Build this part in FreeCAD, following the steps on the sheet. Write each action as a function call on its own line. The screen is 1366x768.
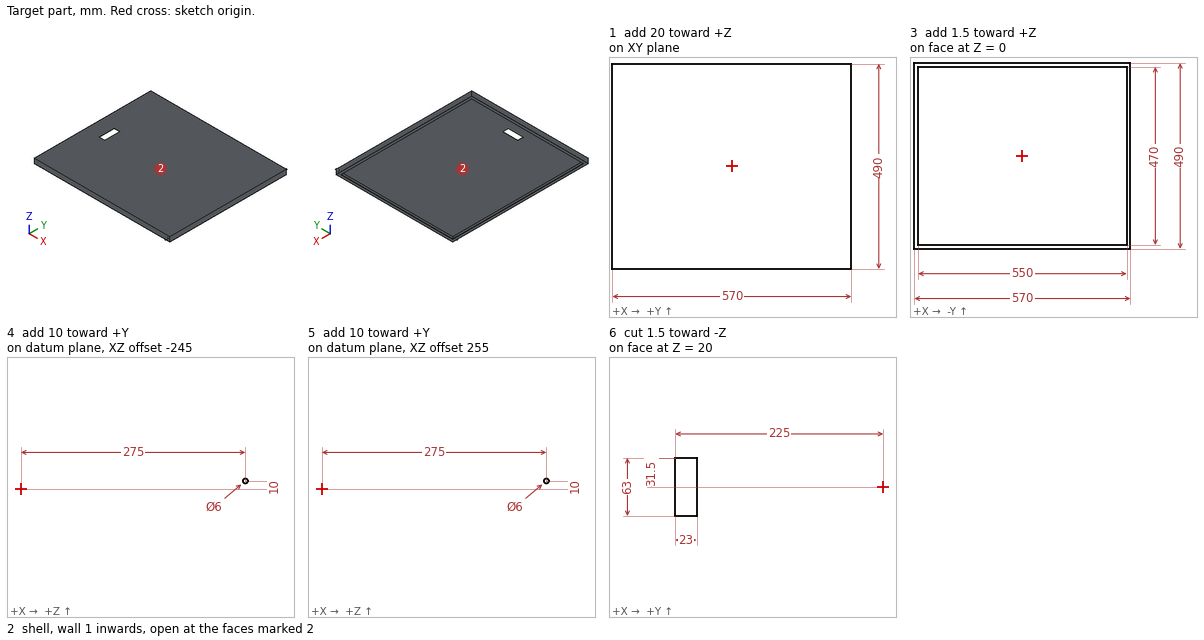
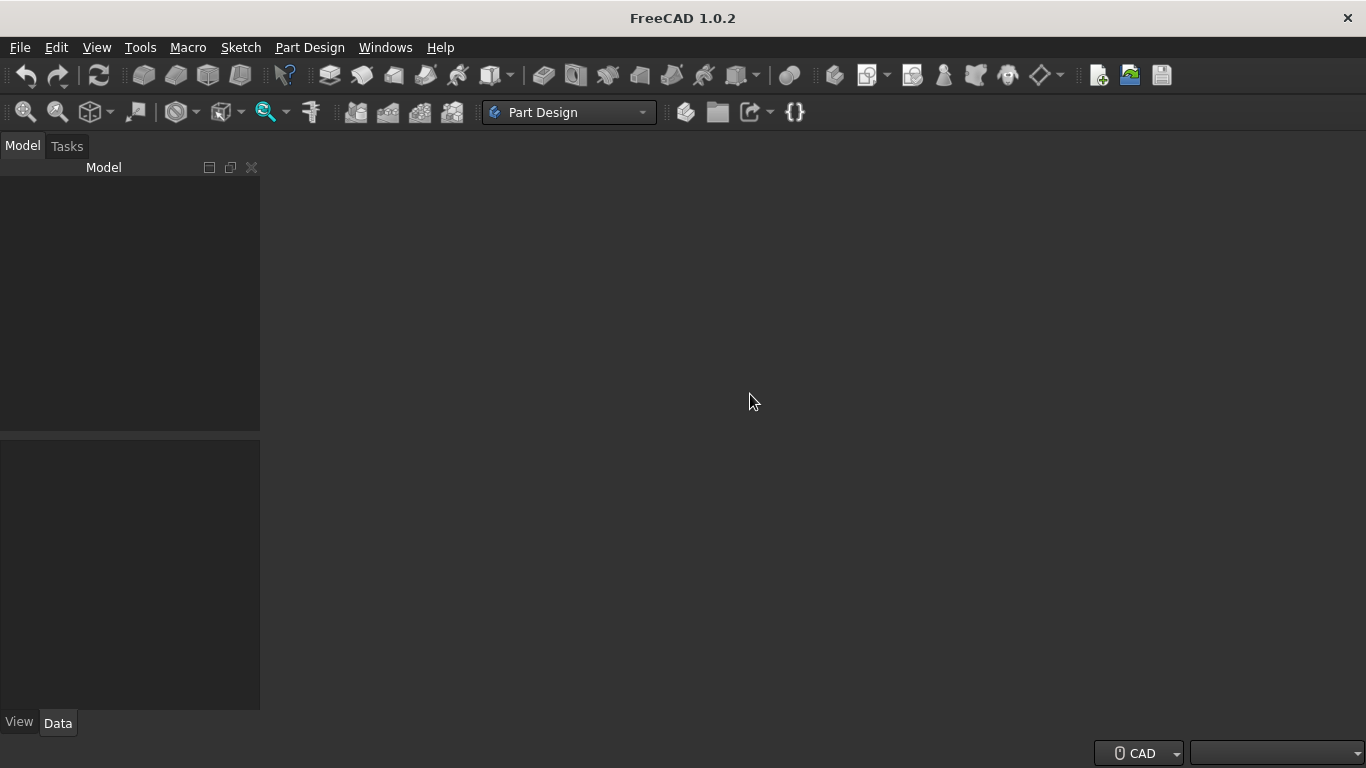
click(1098, 76)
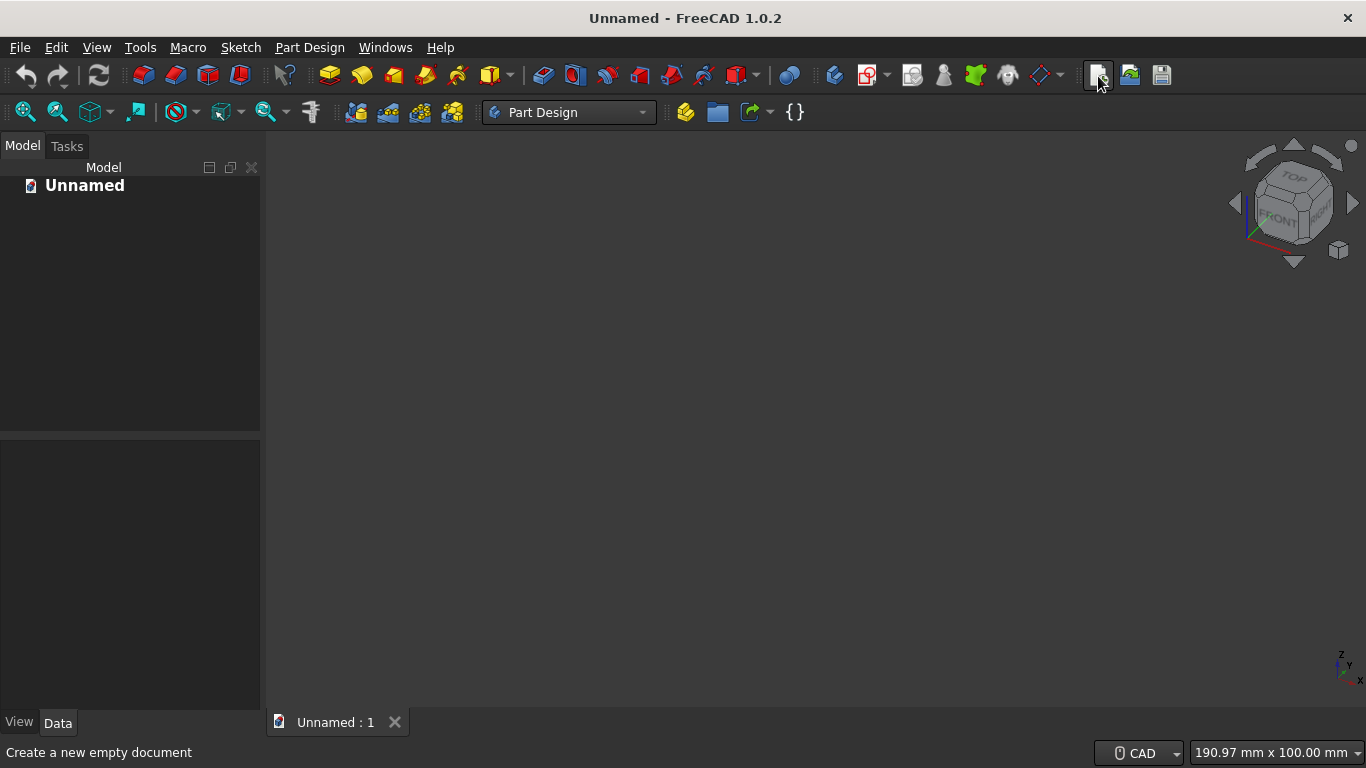
click(868, 76)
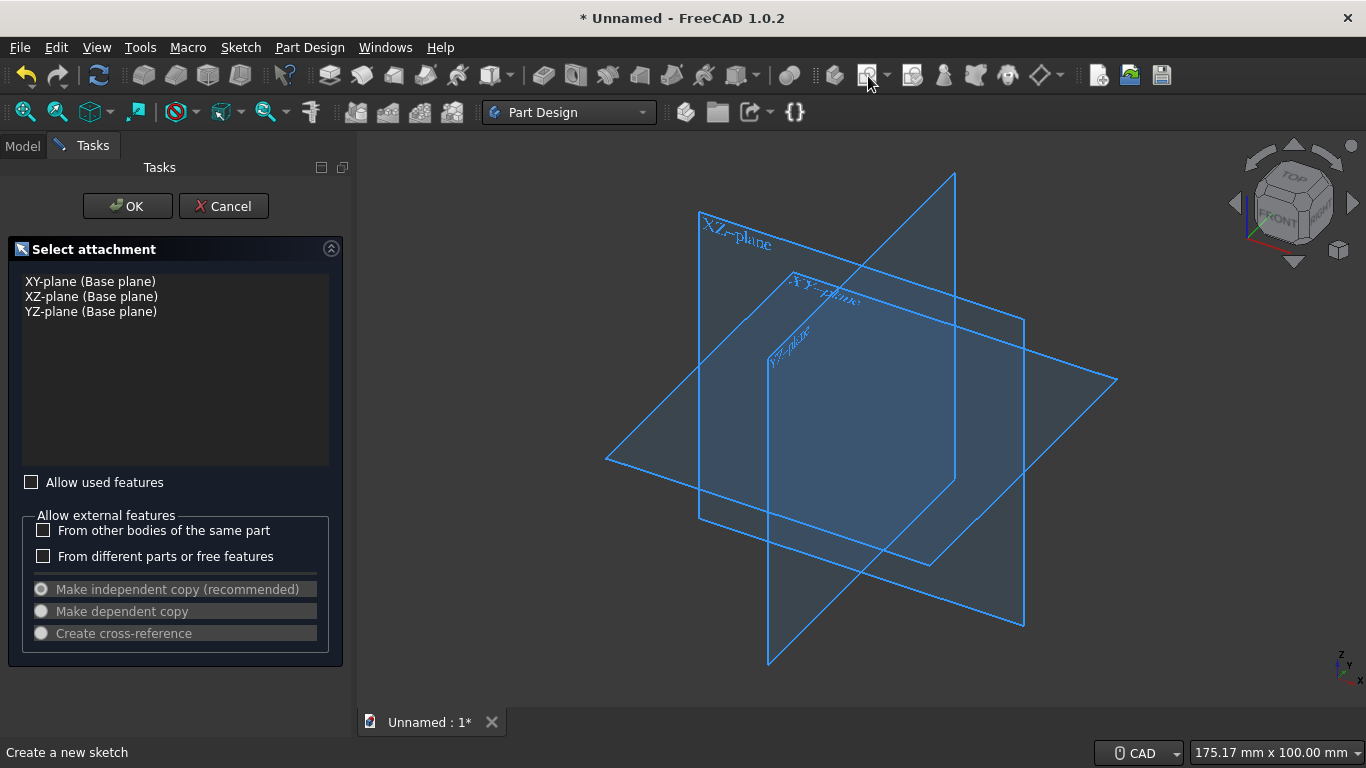
click(82, 282)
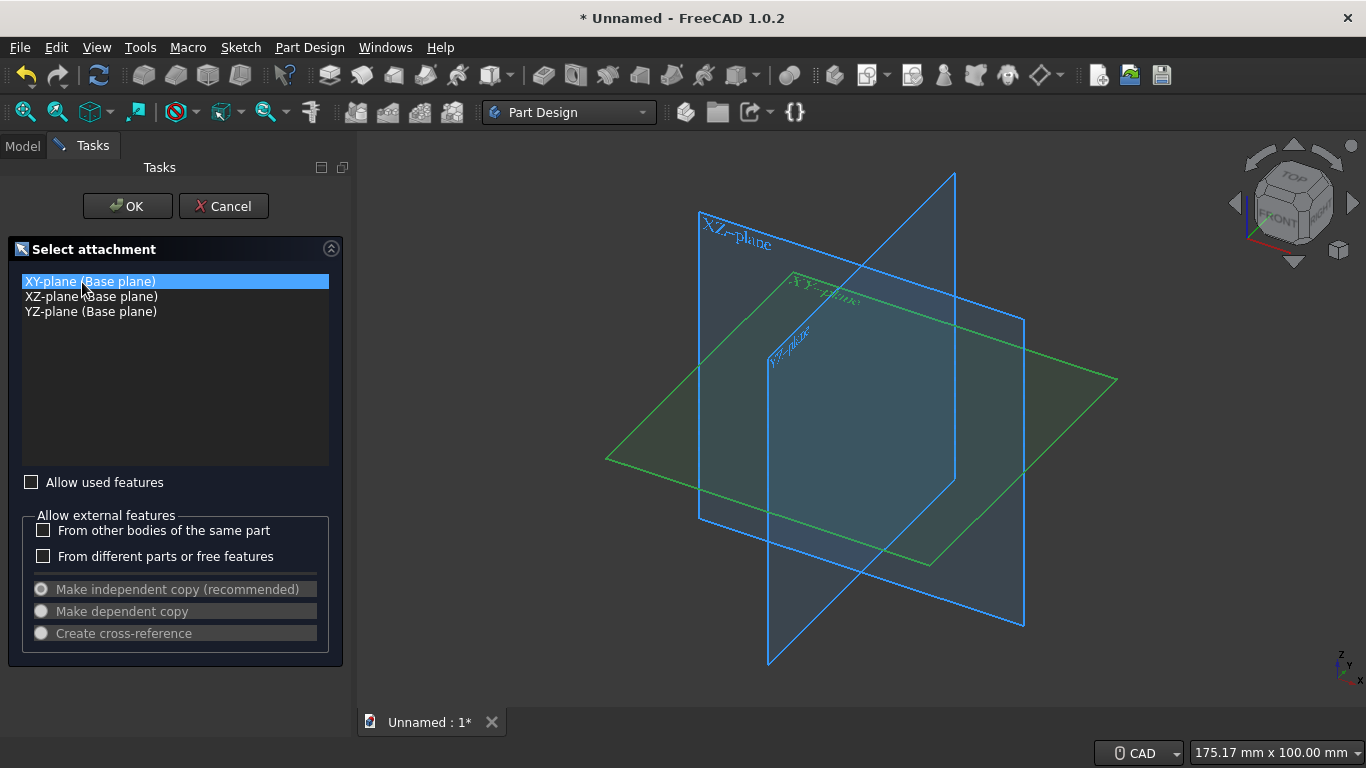
click(128, 206)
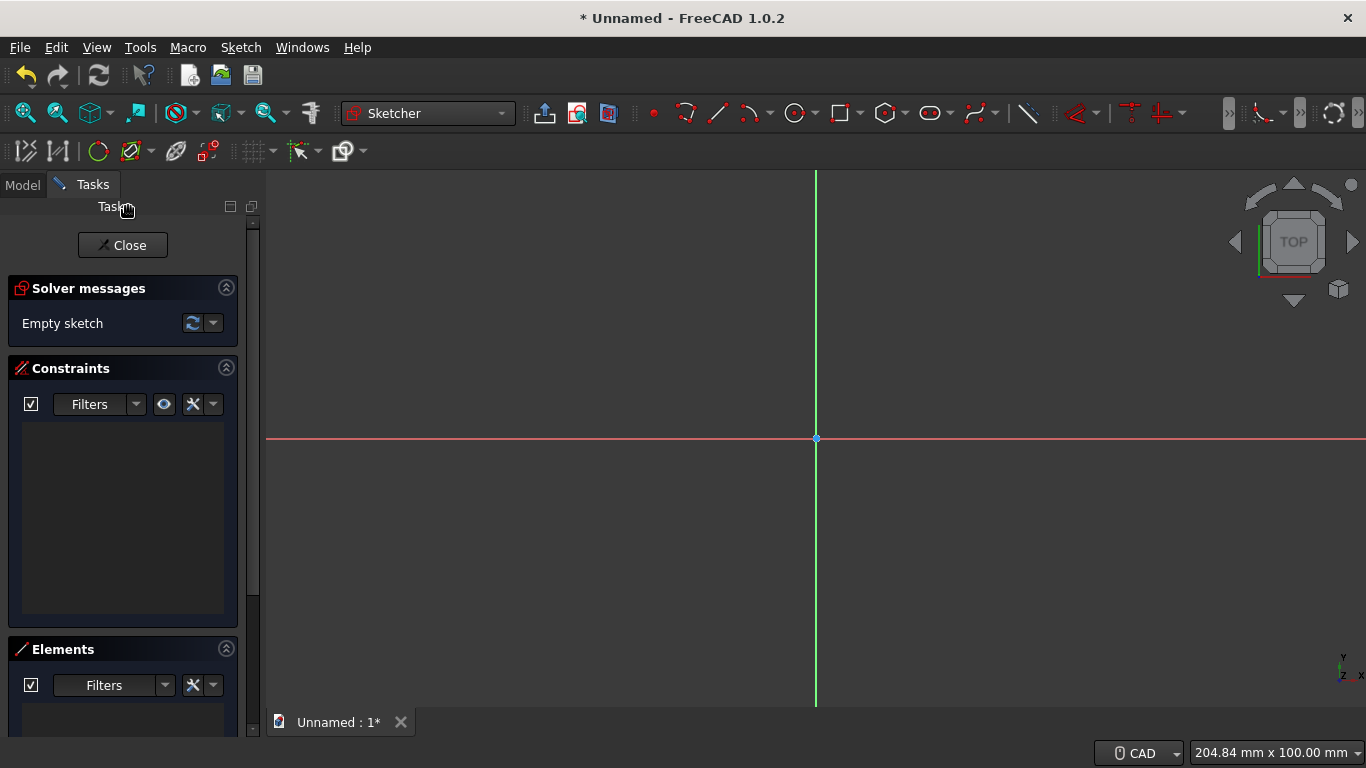
scroll(737, 439, down, 10)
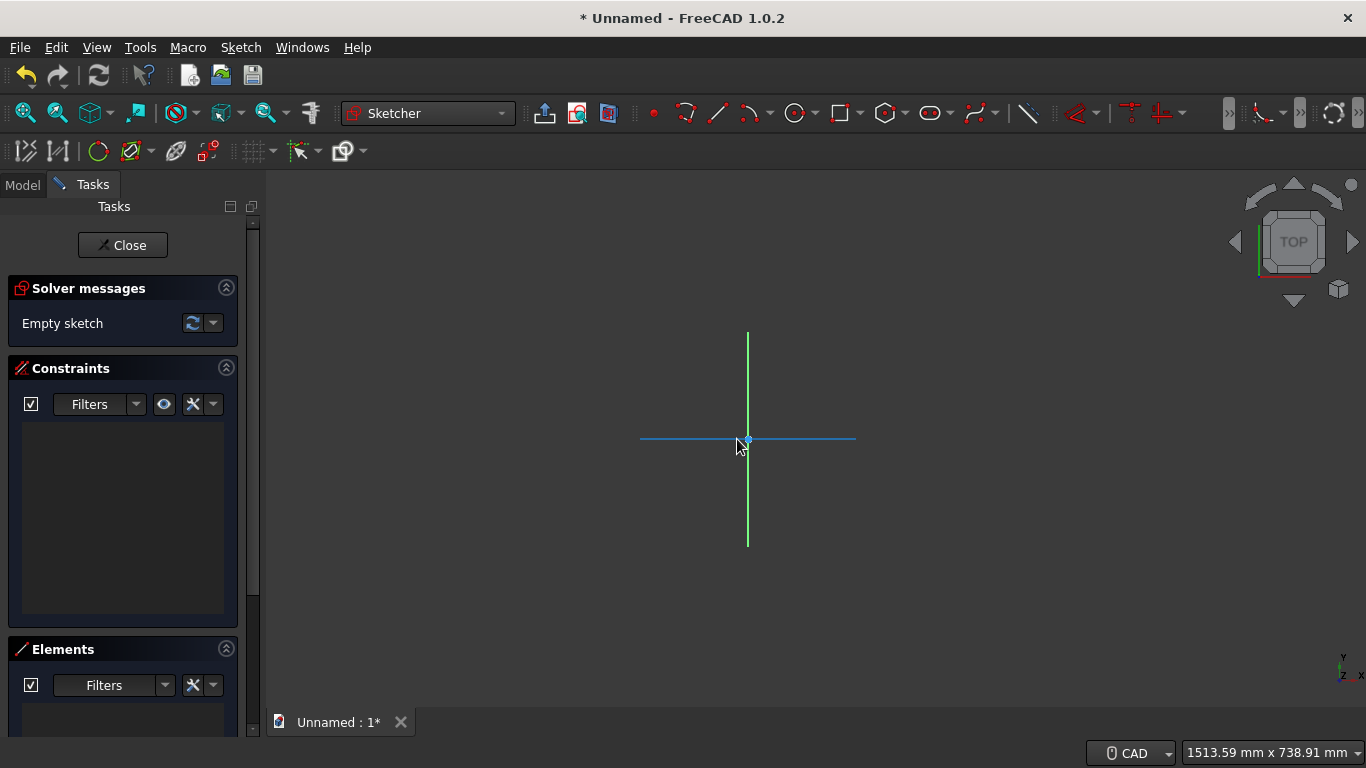
key(g)
key(v)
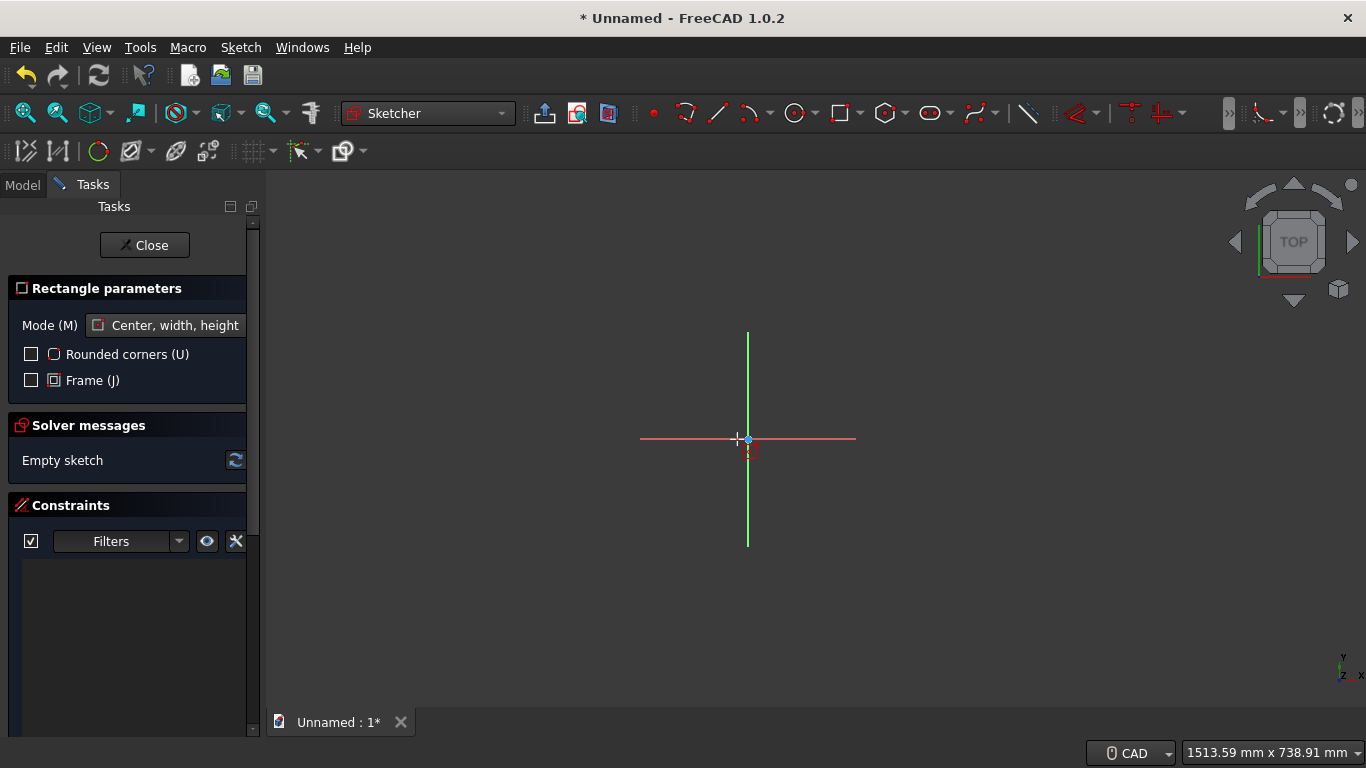
click(748, 439)
click(955, 261)
key(Escape)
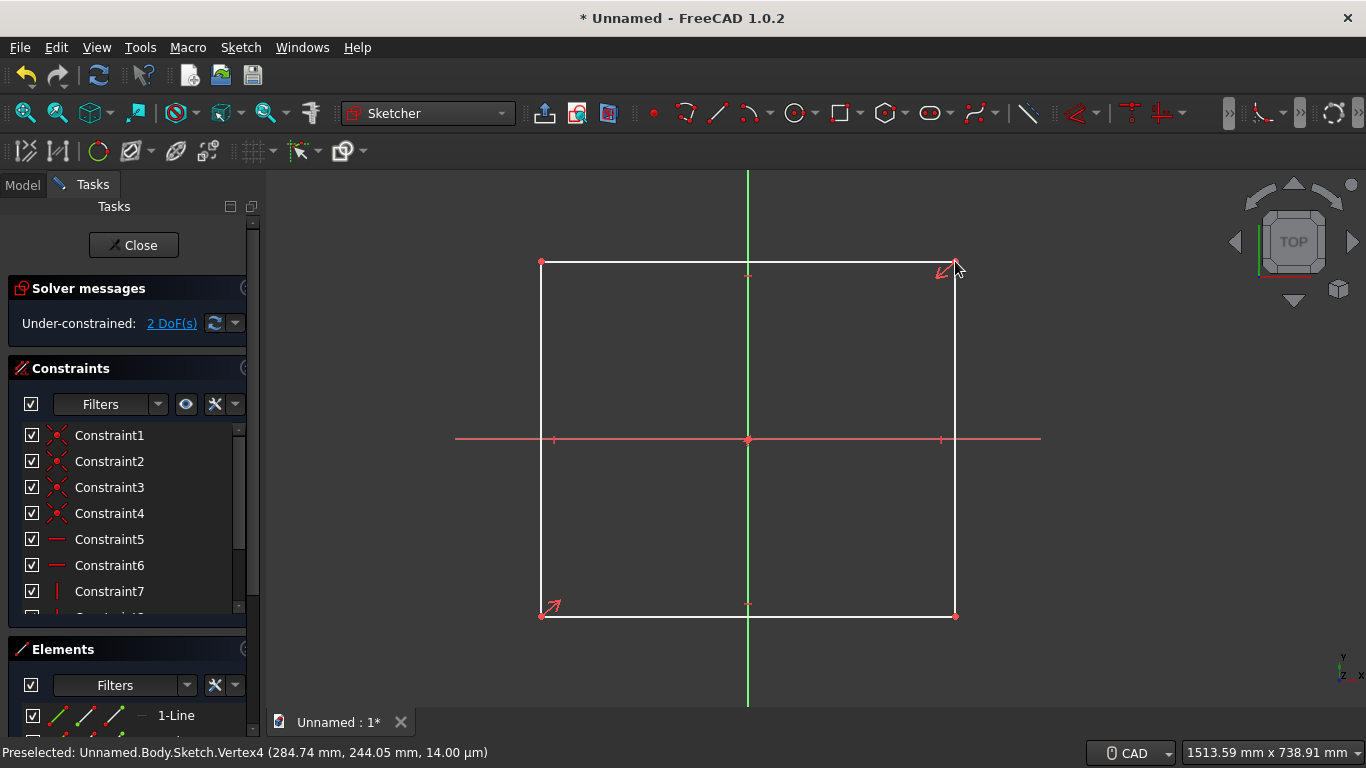
click(665, 617)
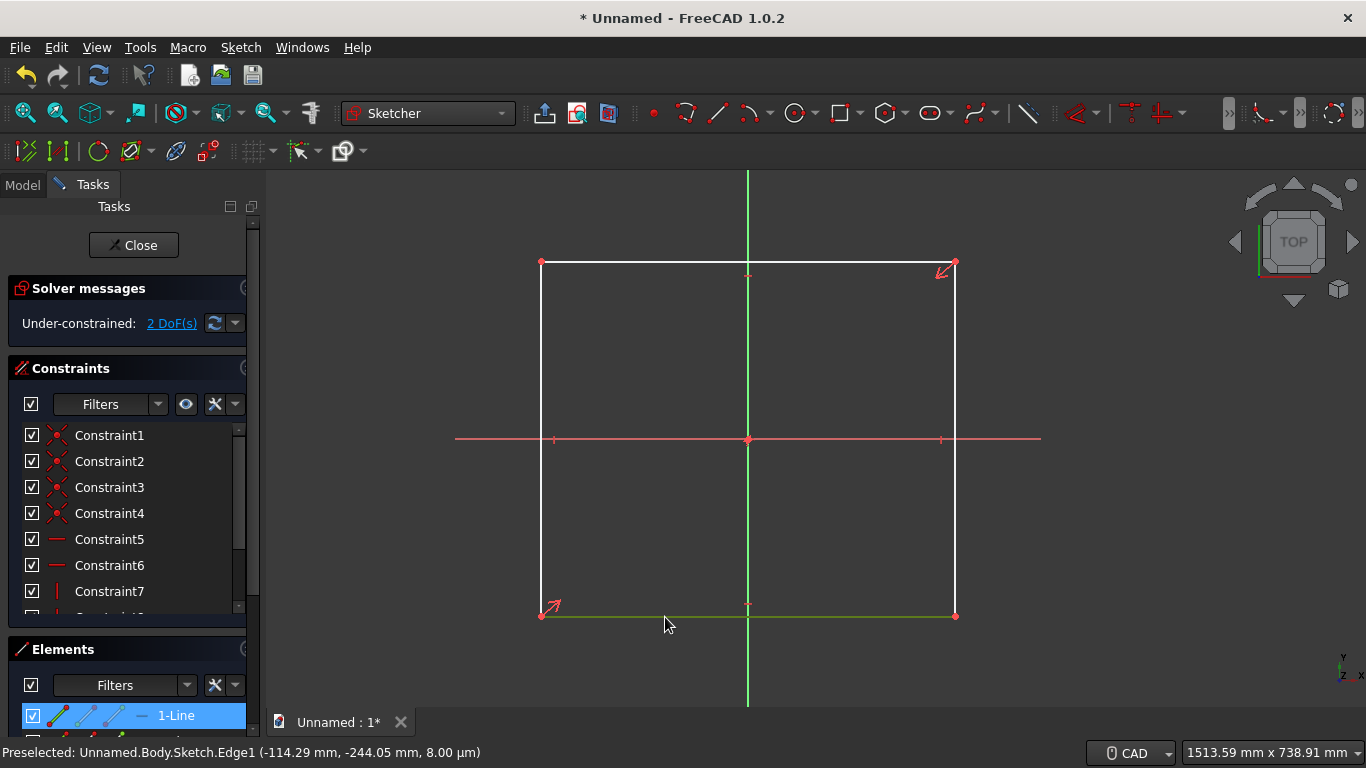
key(l)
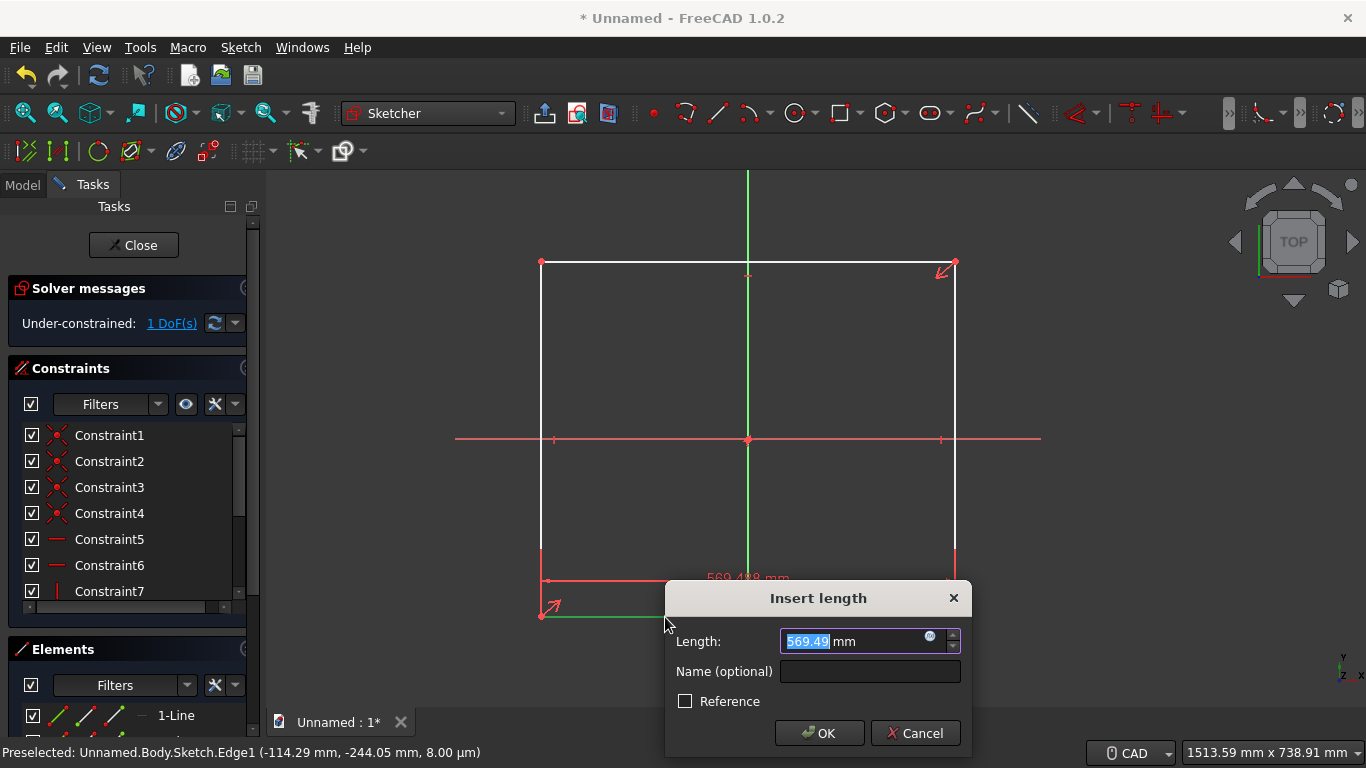
text(570)
key(Return)